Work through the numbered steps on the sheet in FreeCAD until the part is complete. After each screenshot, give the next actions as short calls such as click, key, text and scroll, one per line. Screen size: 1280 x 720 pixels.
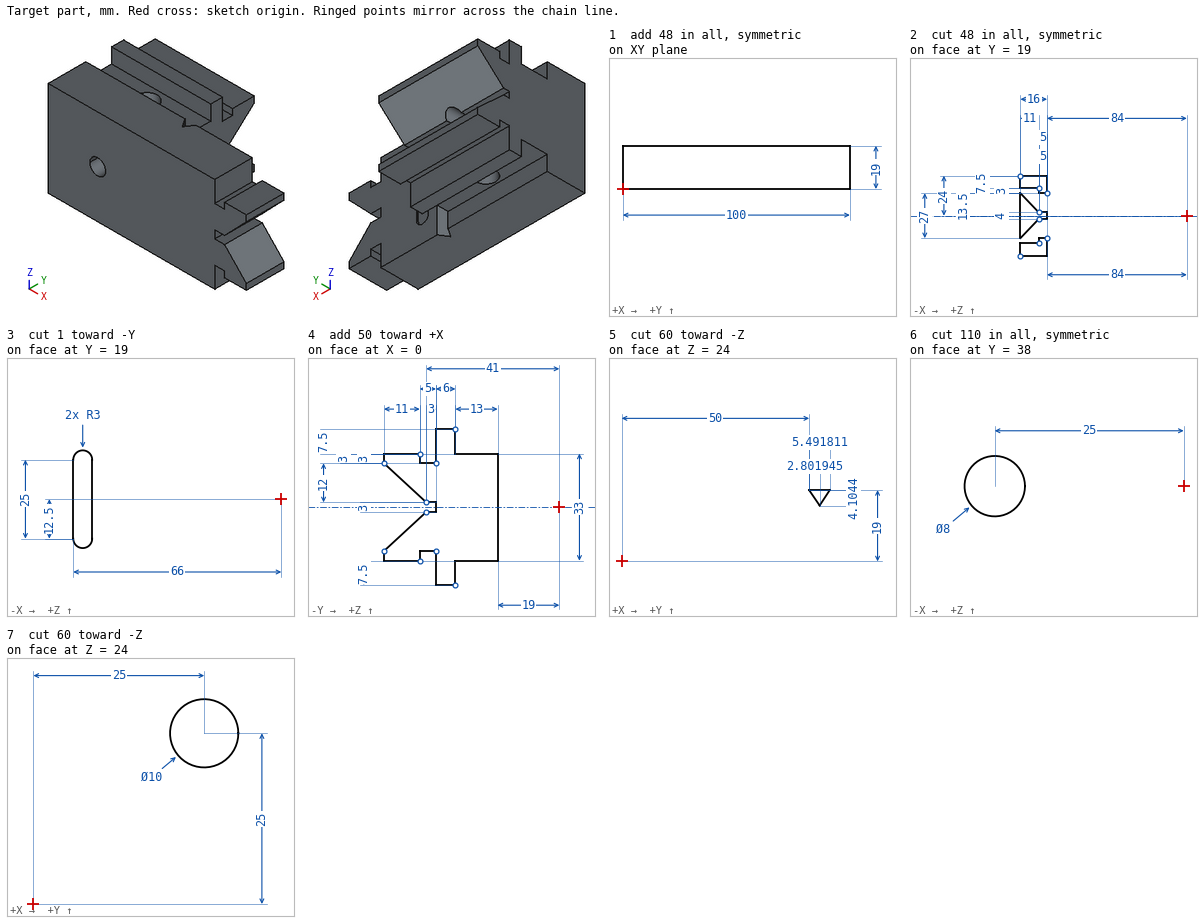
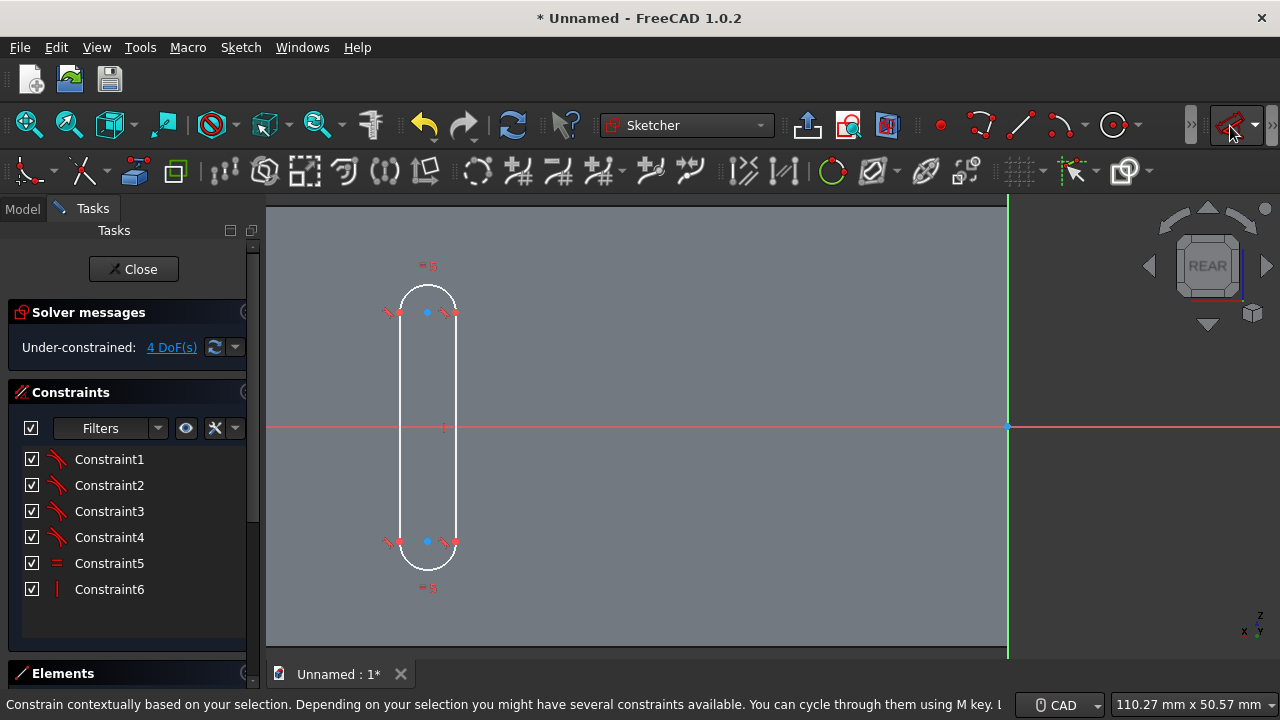
scroll(412, 565, up, 2)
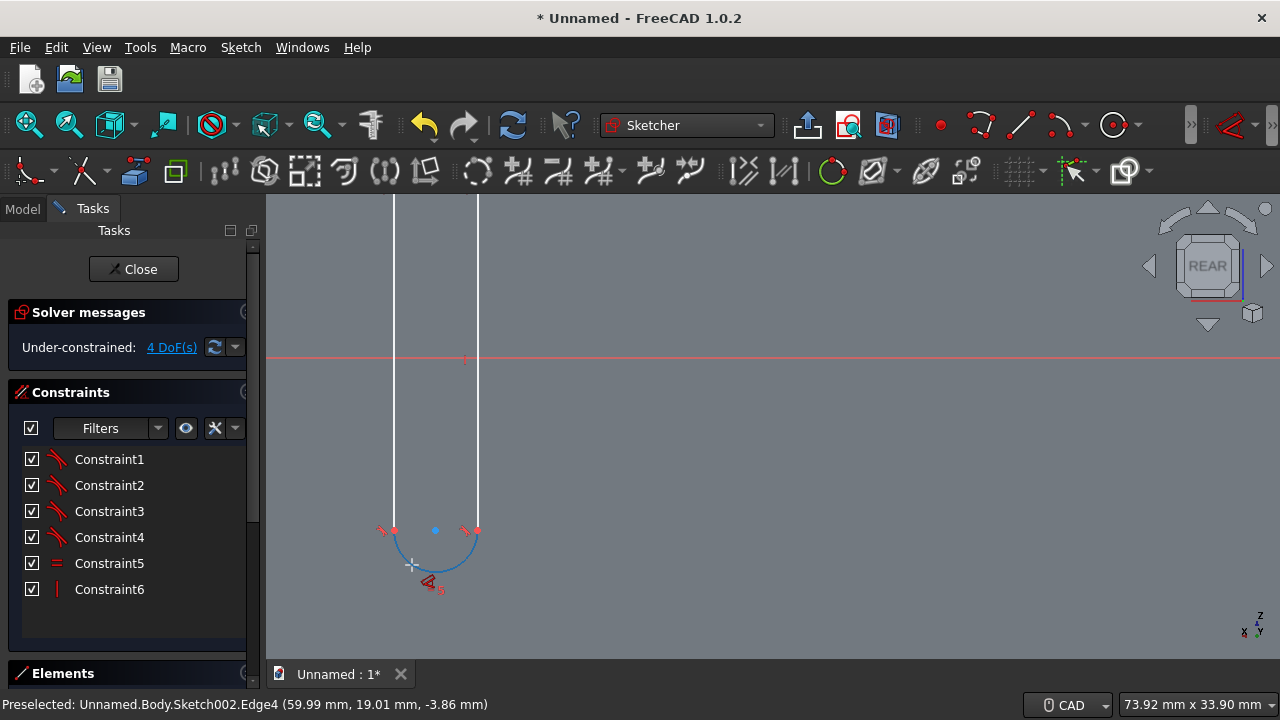
click(411, 564)
click(392, 590)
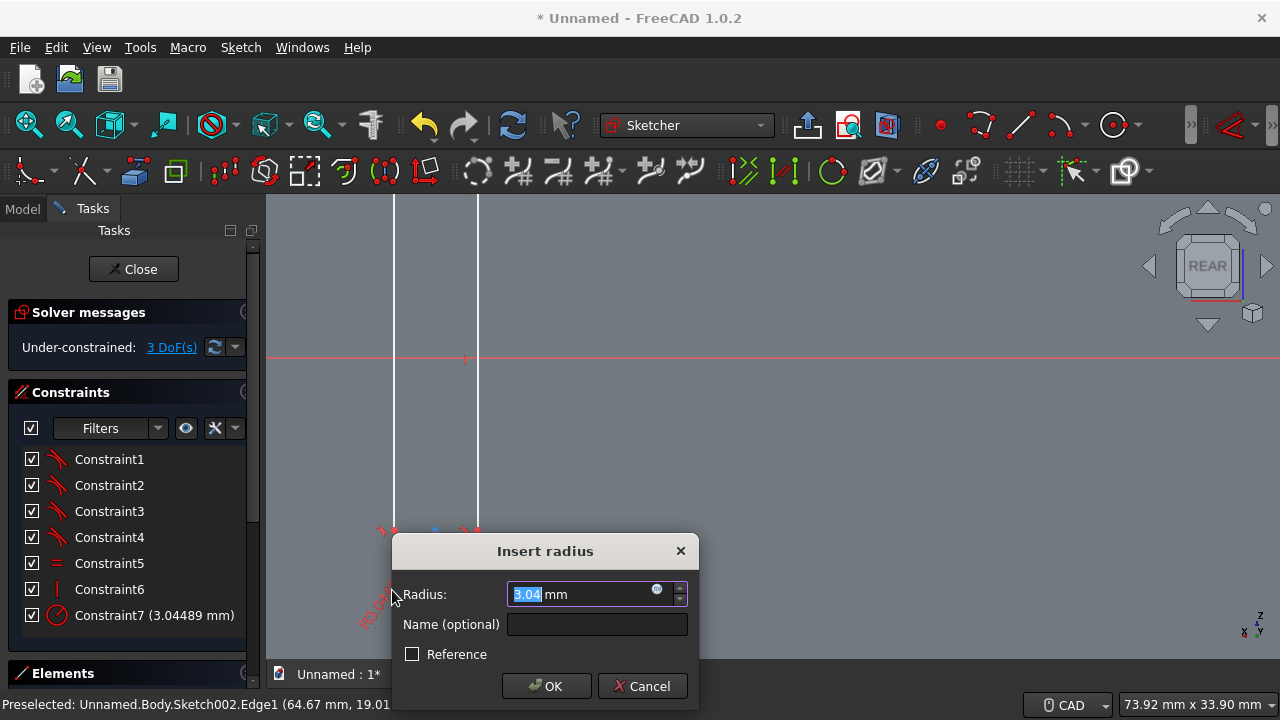
text(3)
key(Return)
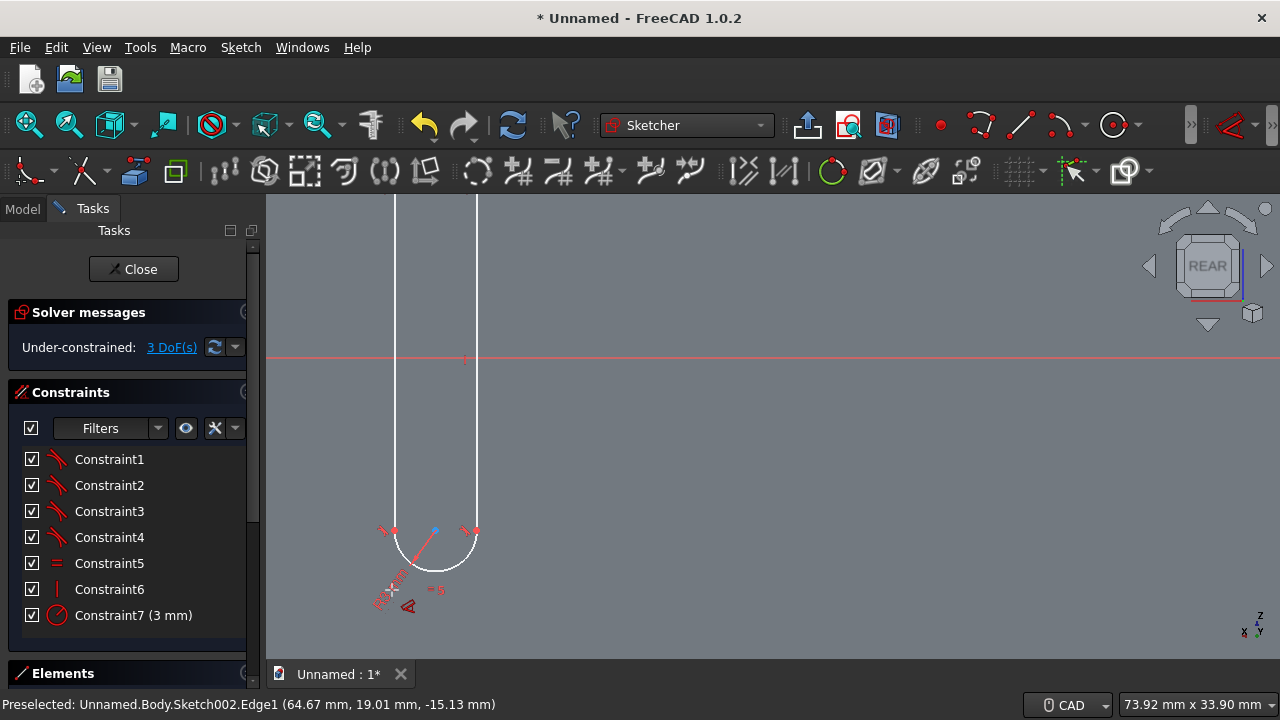
click(395, 428)
click(361, 376)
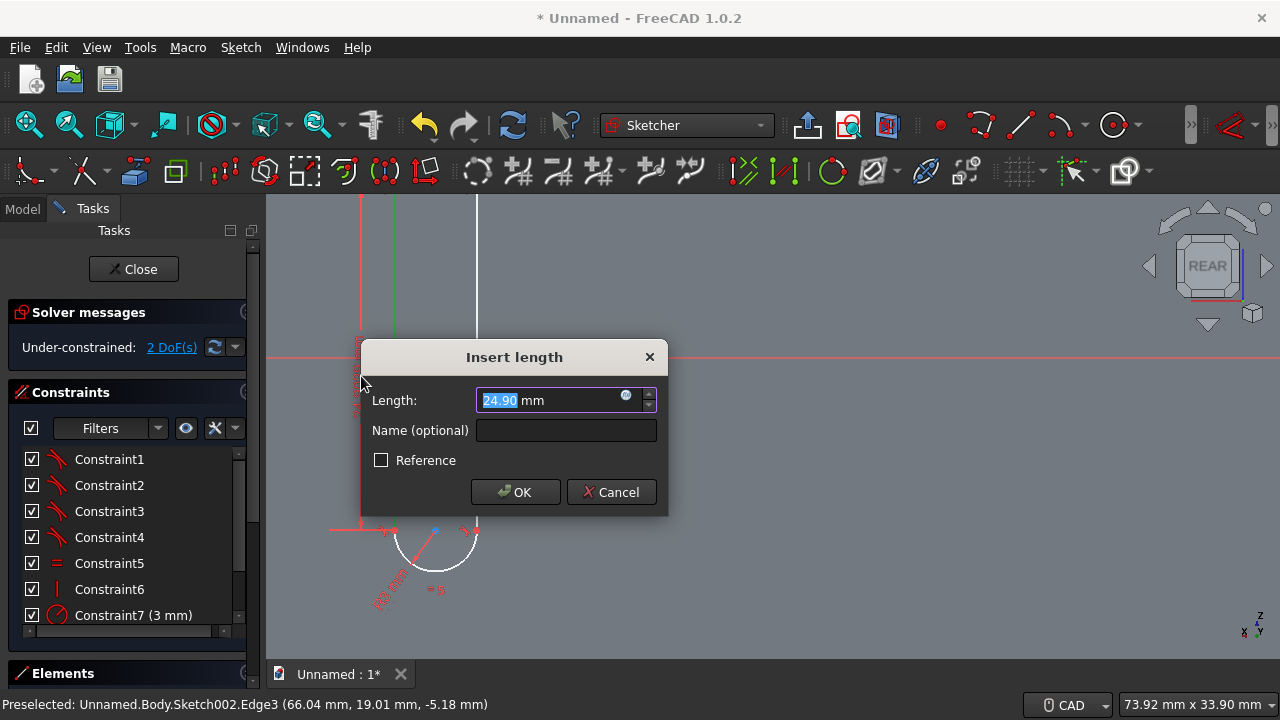
text(25)
key(Return)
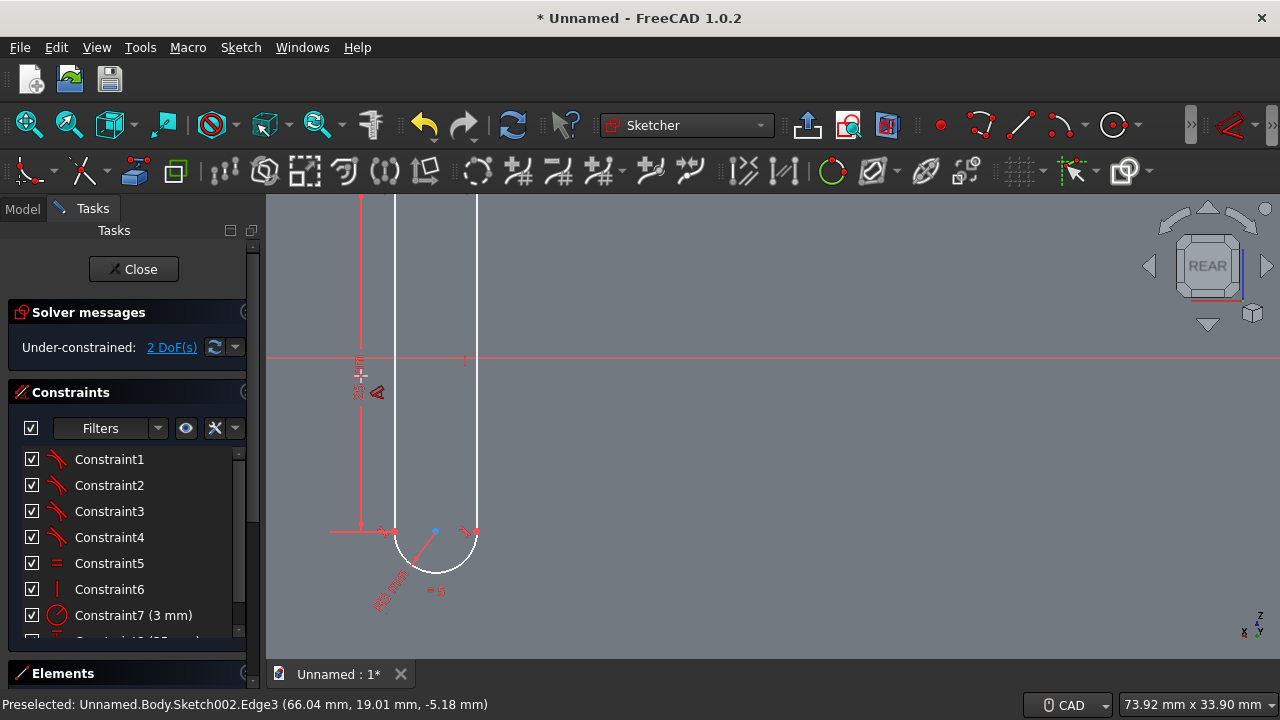
click(395, 532)
click(755, 566)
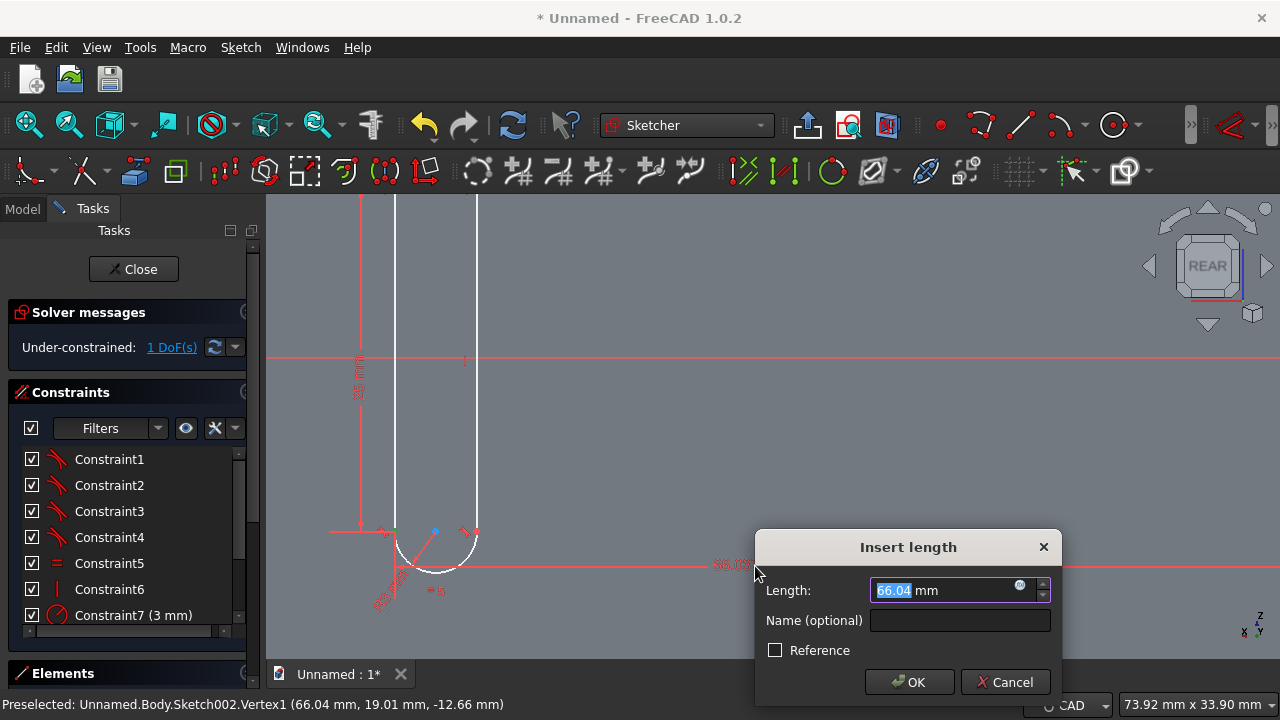
text(66)
key(Return)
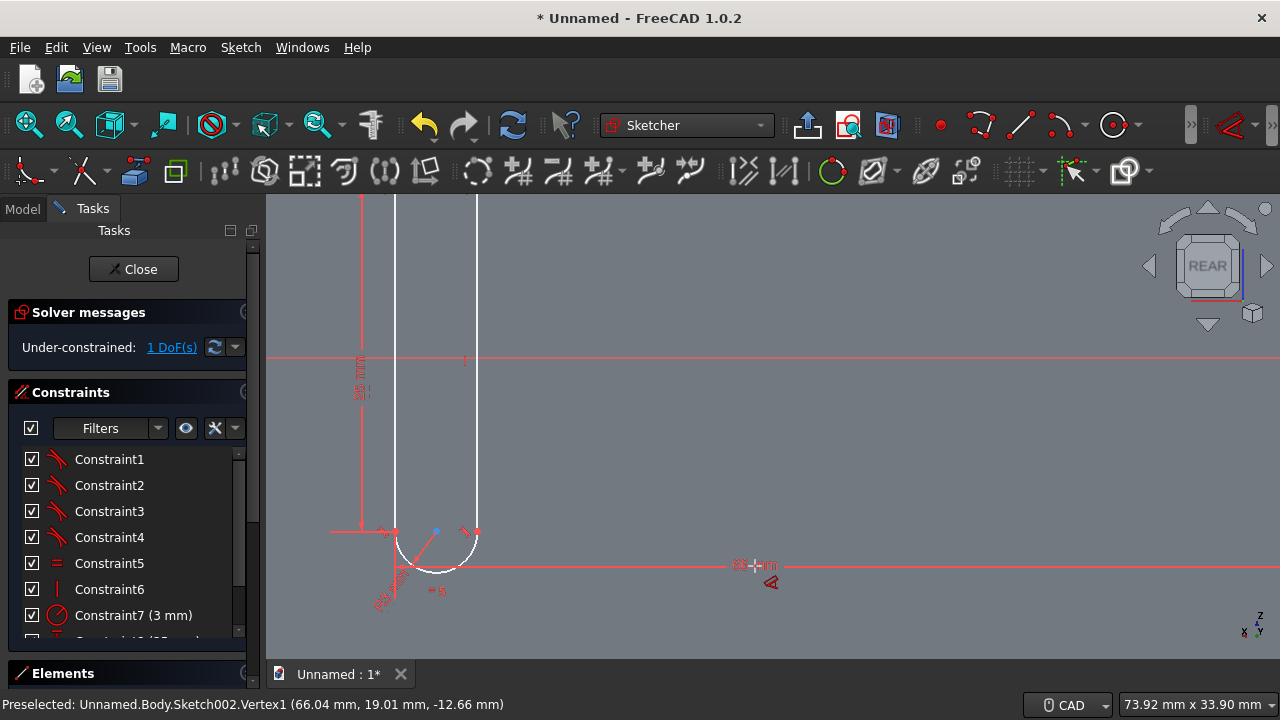
click(395, 532)
click(361, 445)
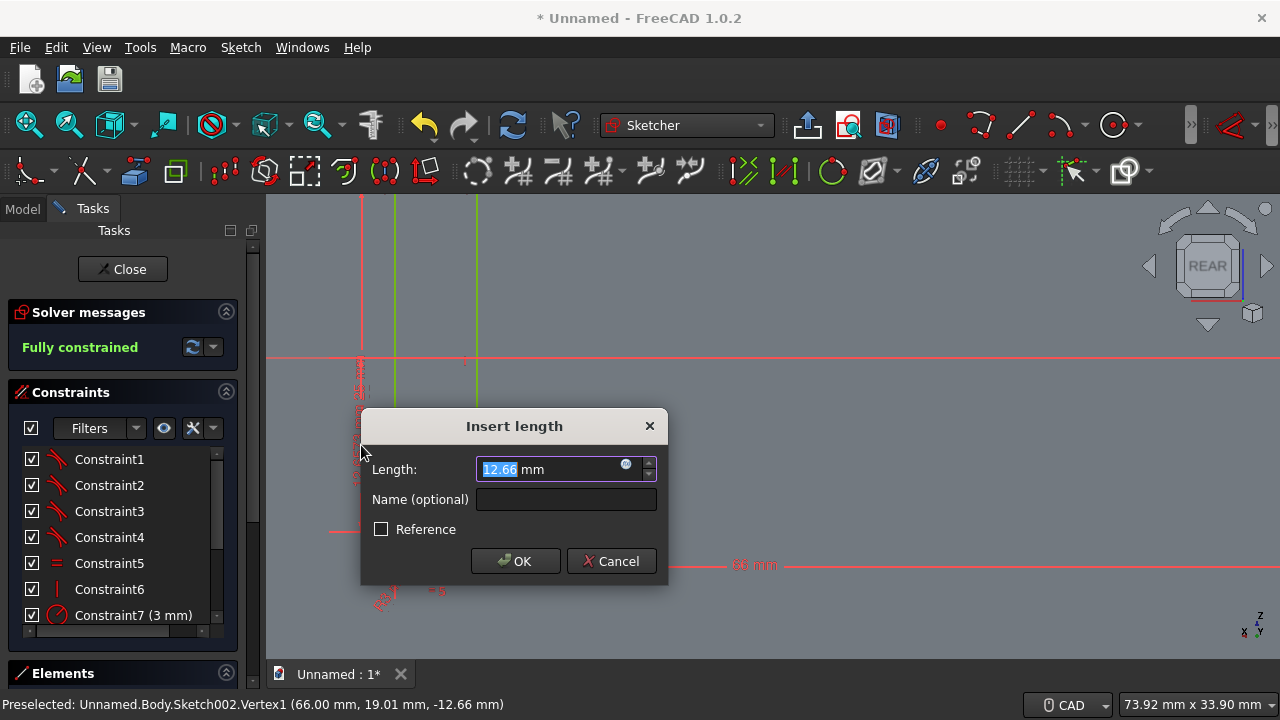
text(12.5)
key(Return)
key(Escape)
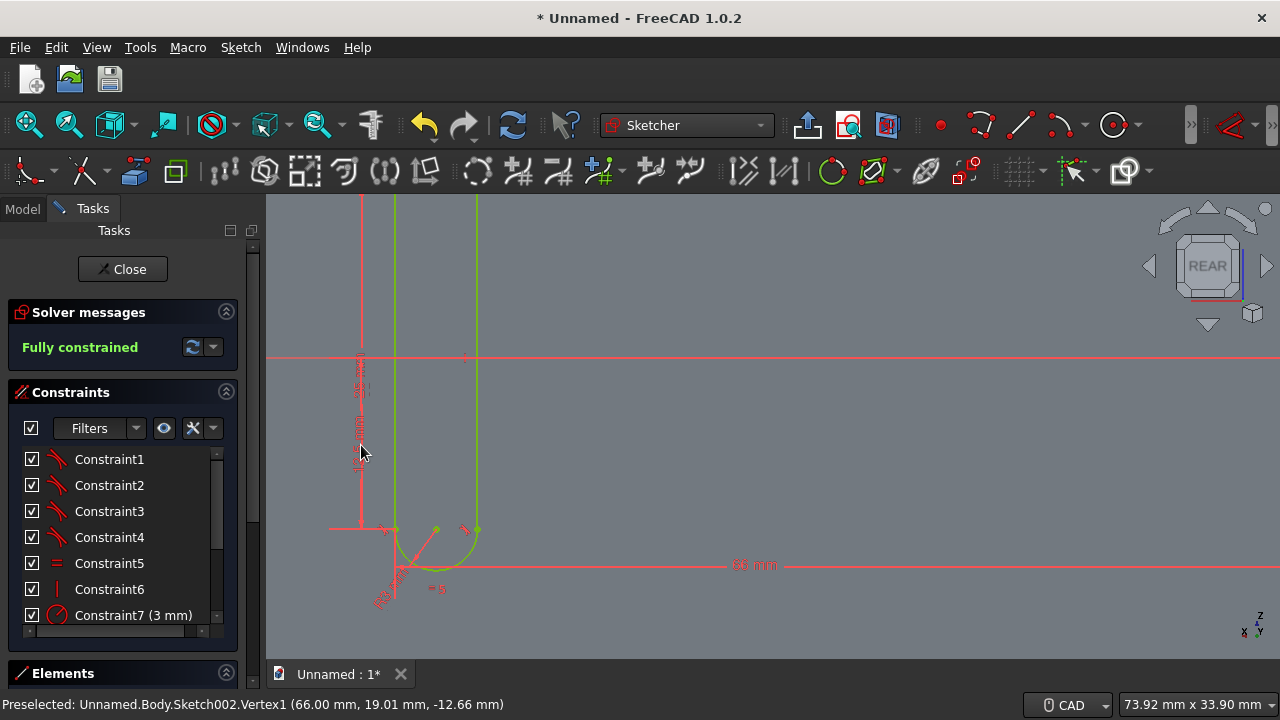
click(123, 269)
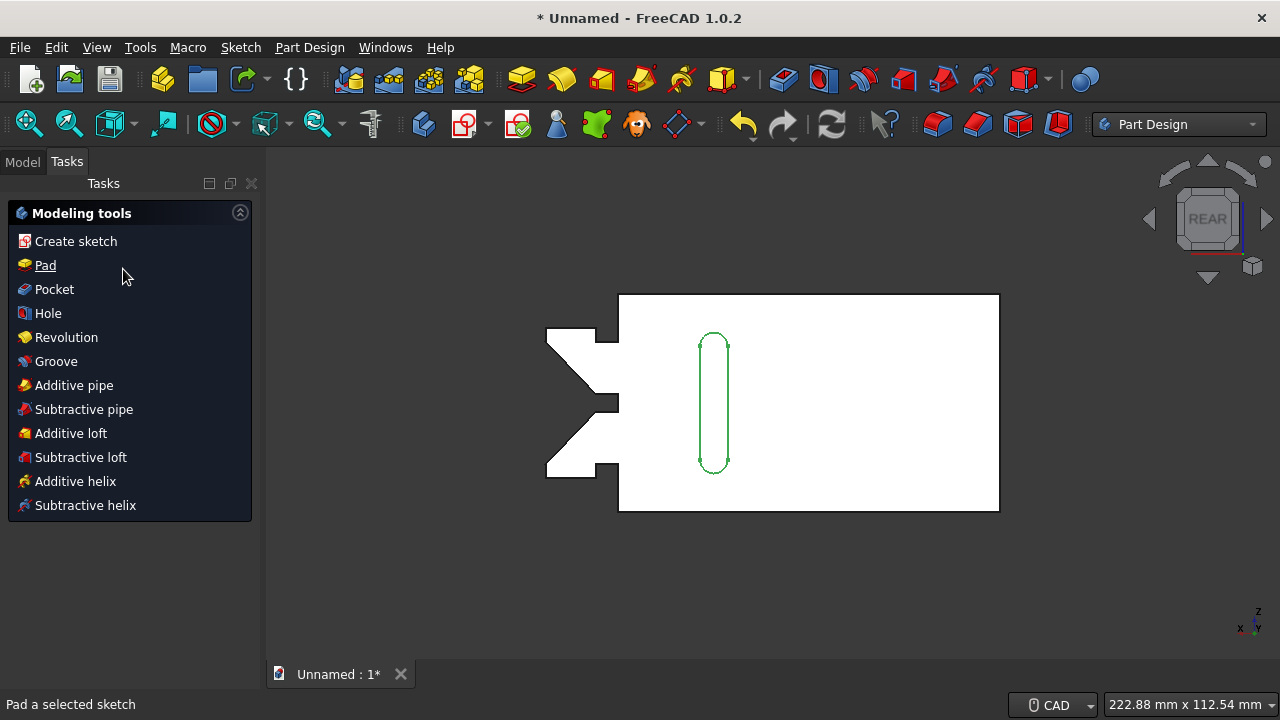
click(784, 80)